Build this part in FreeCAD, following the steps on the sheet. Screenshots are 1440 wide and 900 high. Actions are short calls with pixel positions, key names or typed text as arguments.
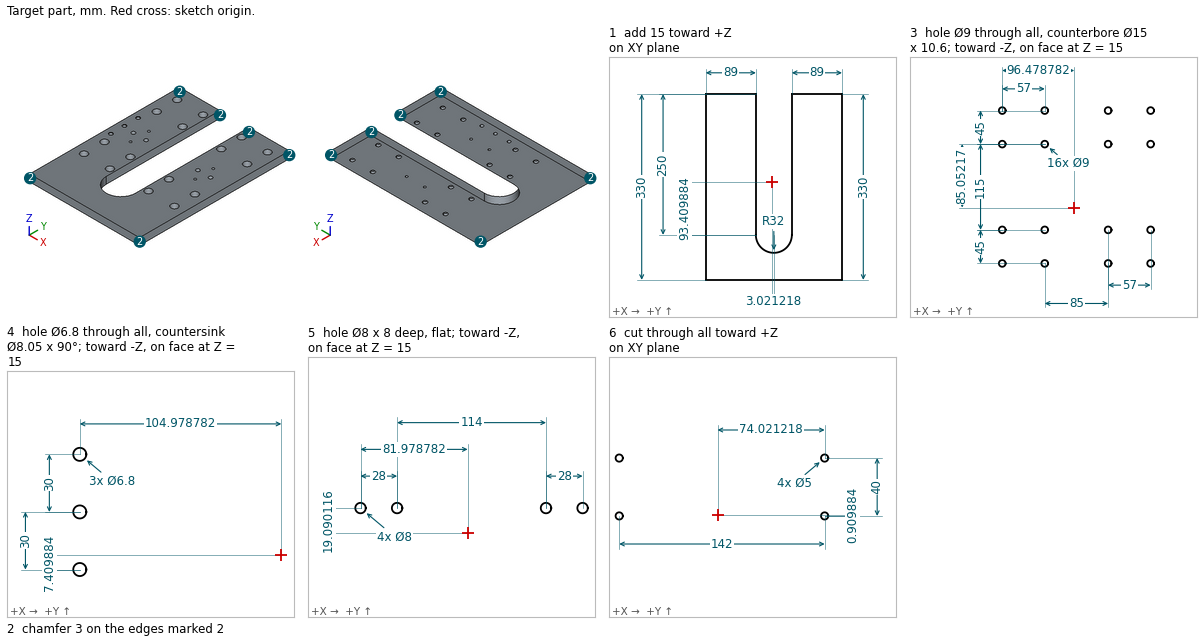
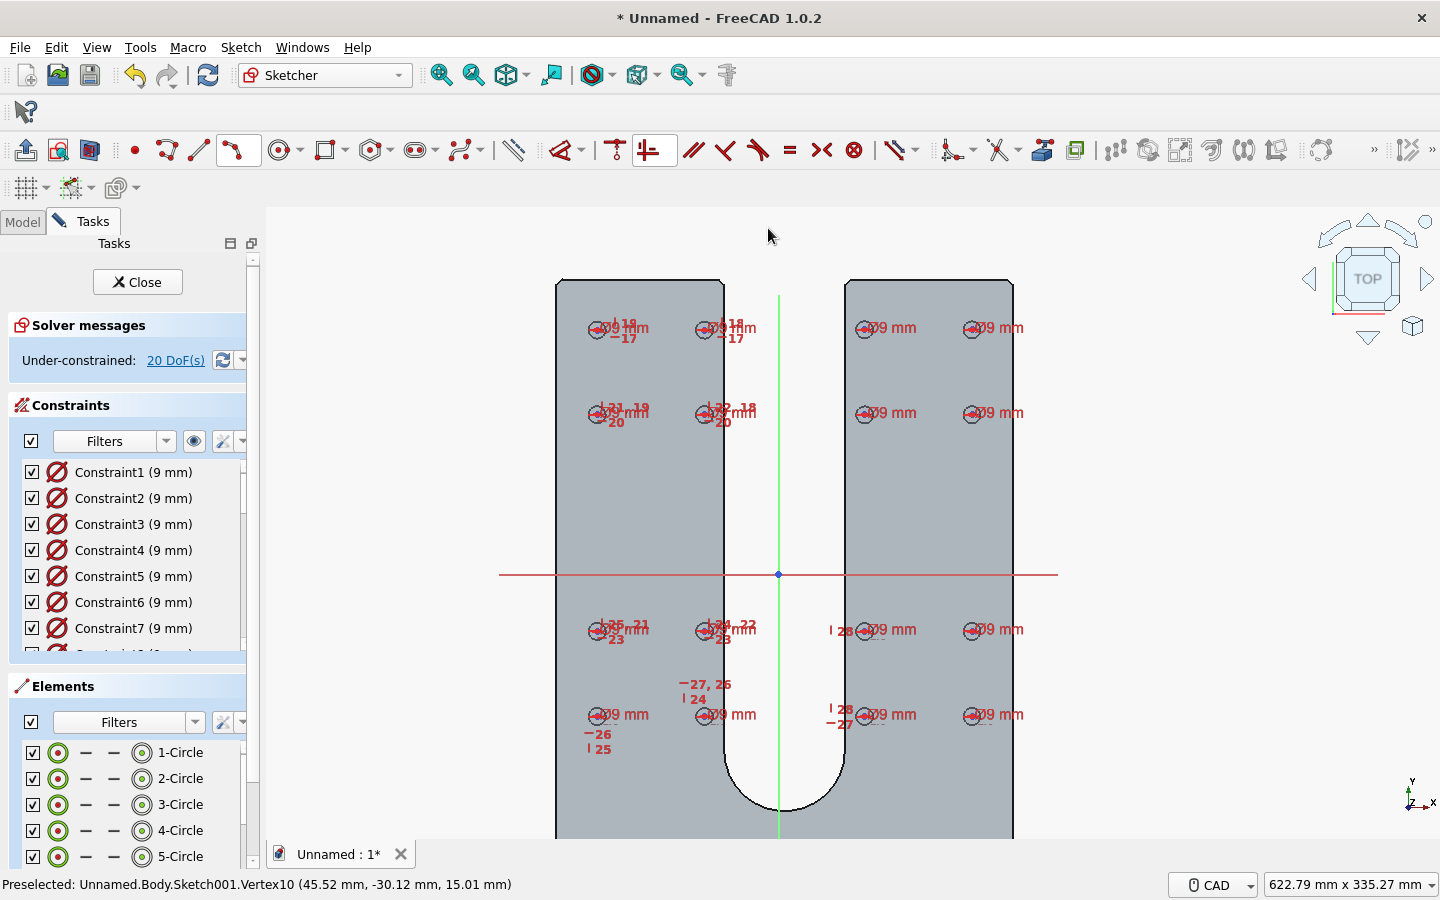
click(705, 631)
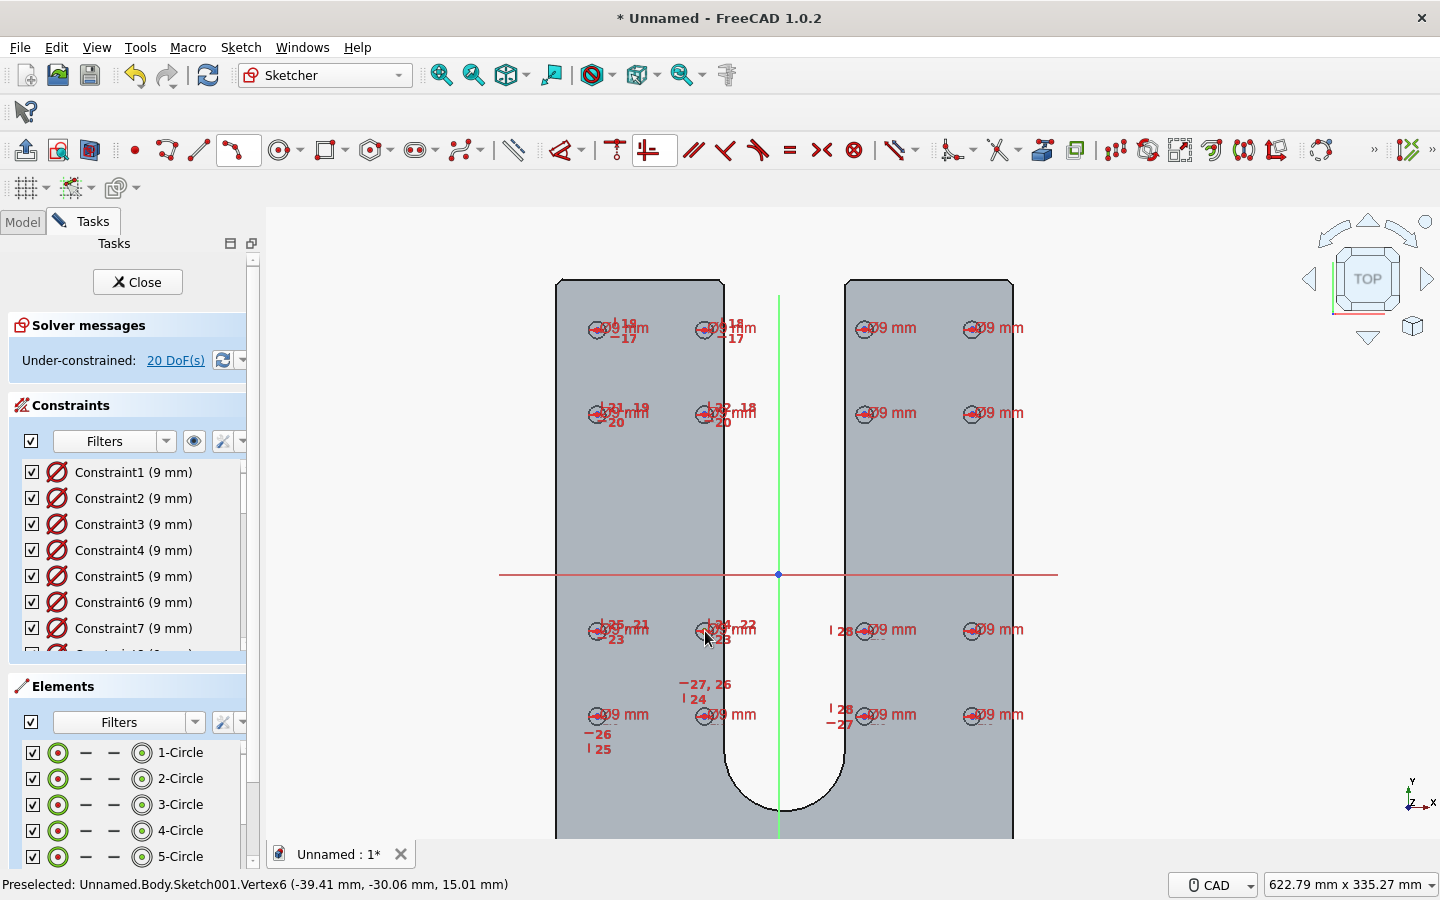
click(865, 632)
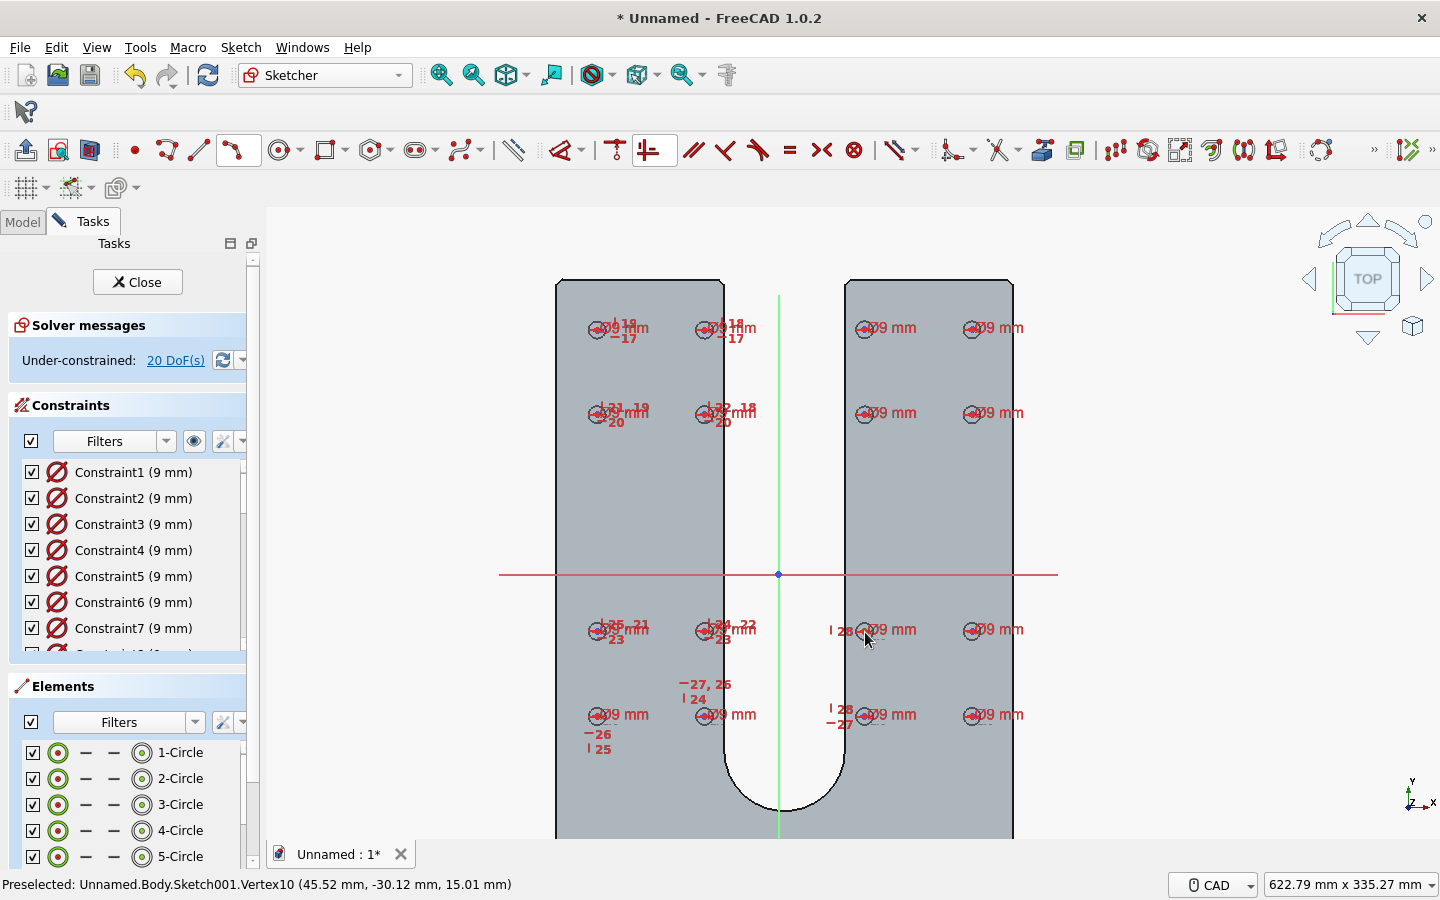
key(h)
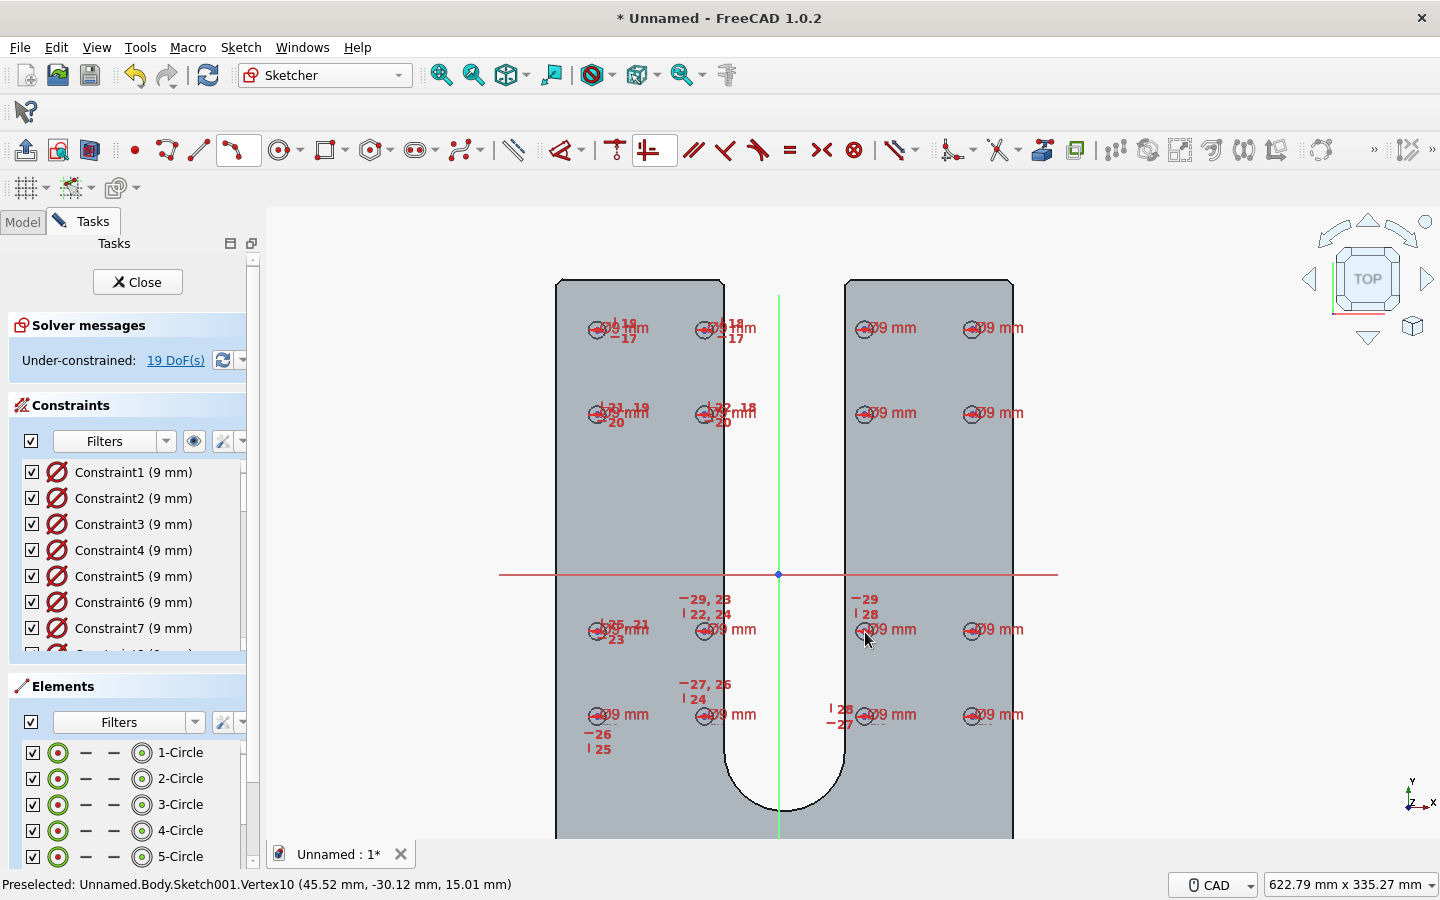
click(865, 631)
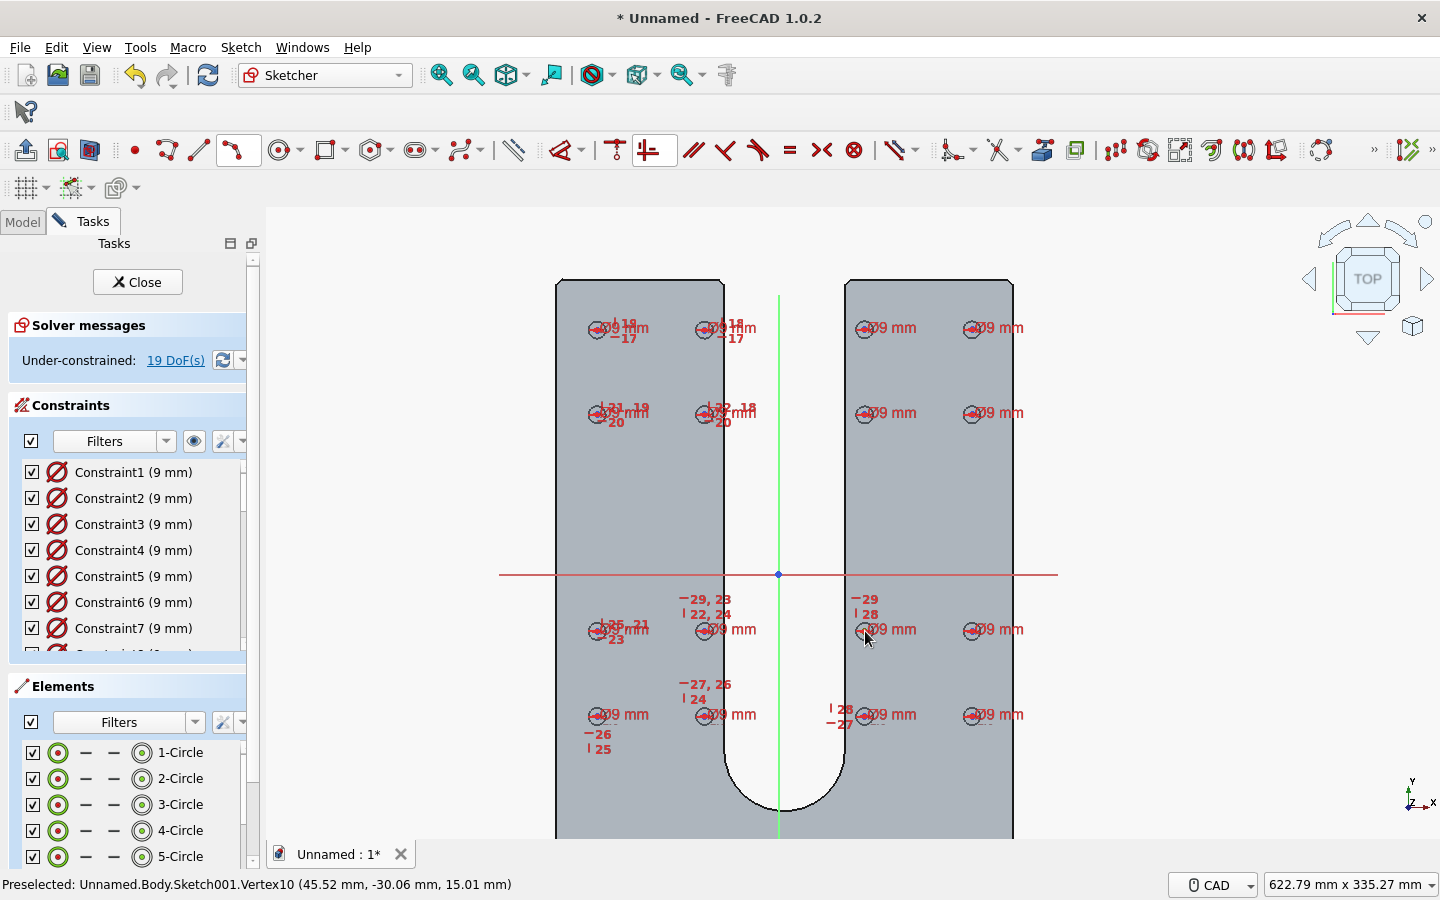
click(972, 631)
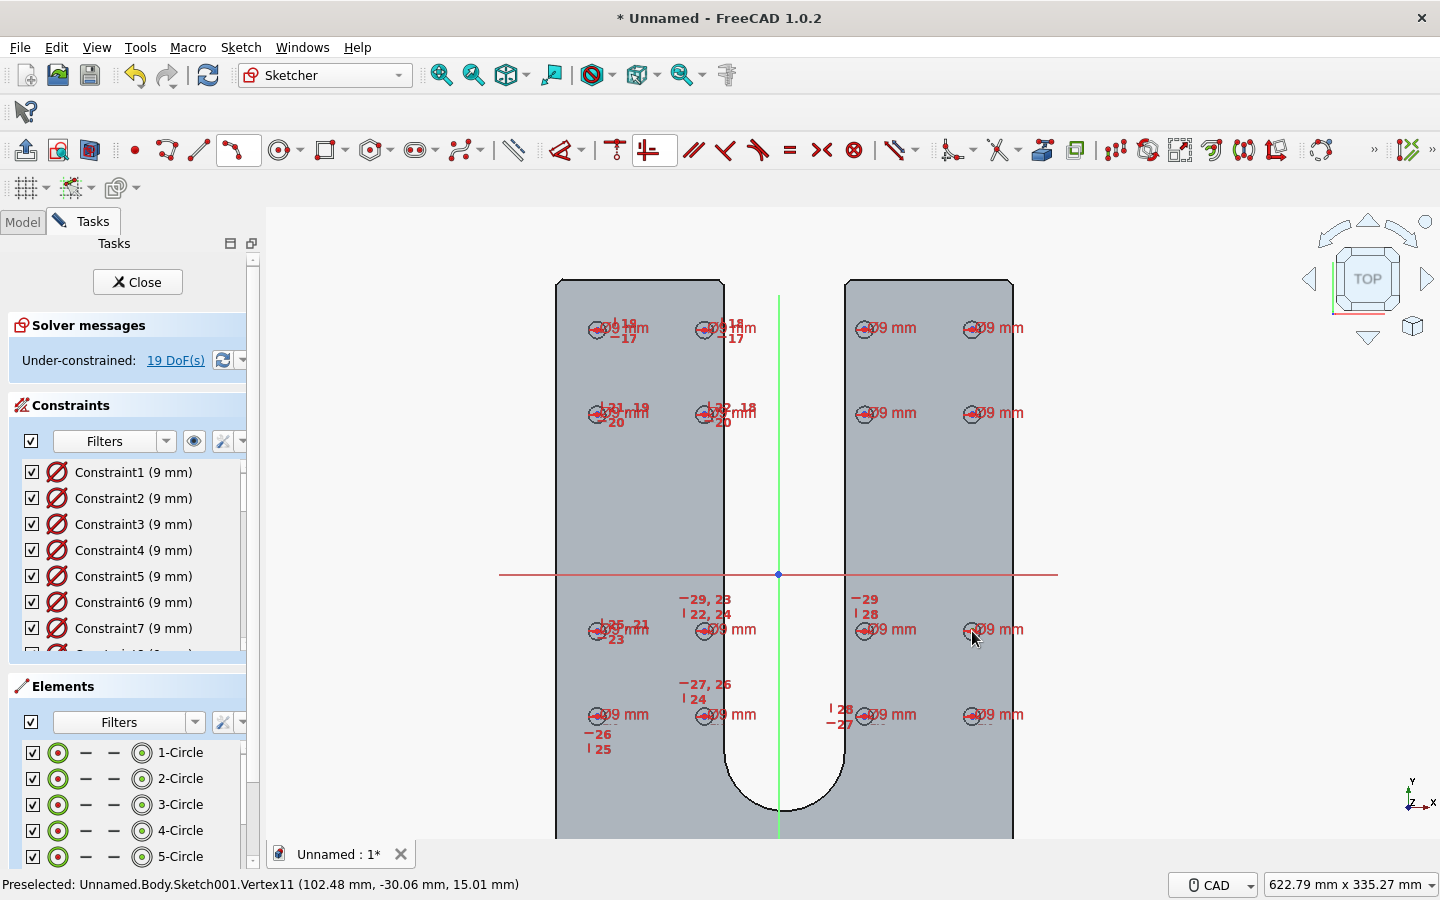
click(672, 150)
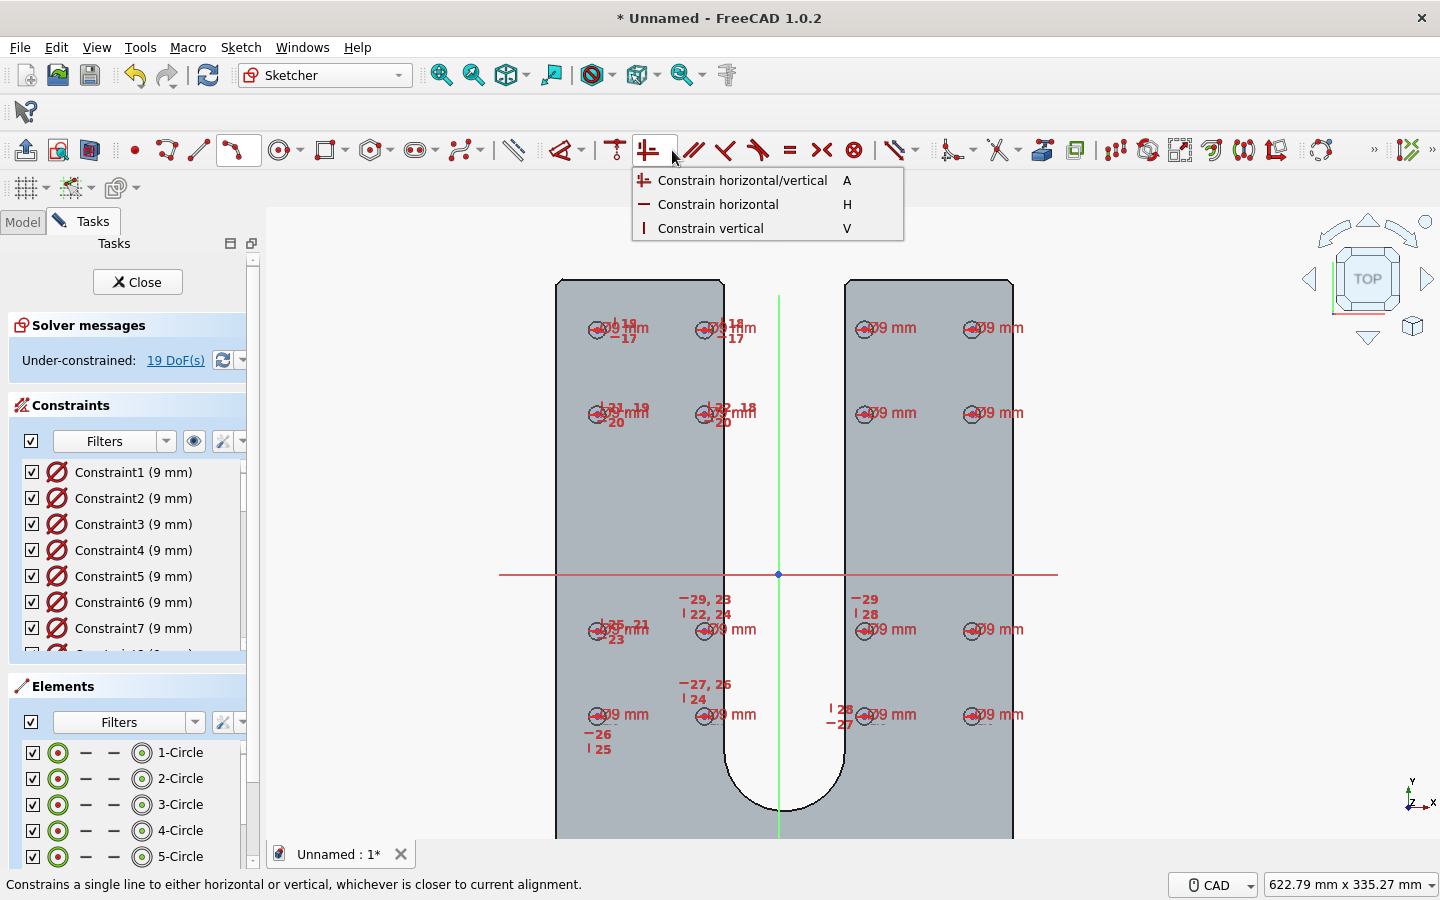
click(768, 204)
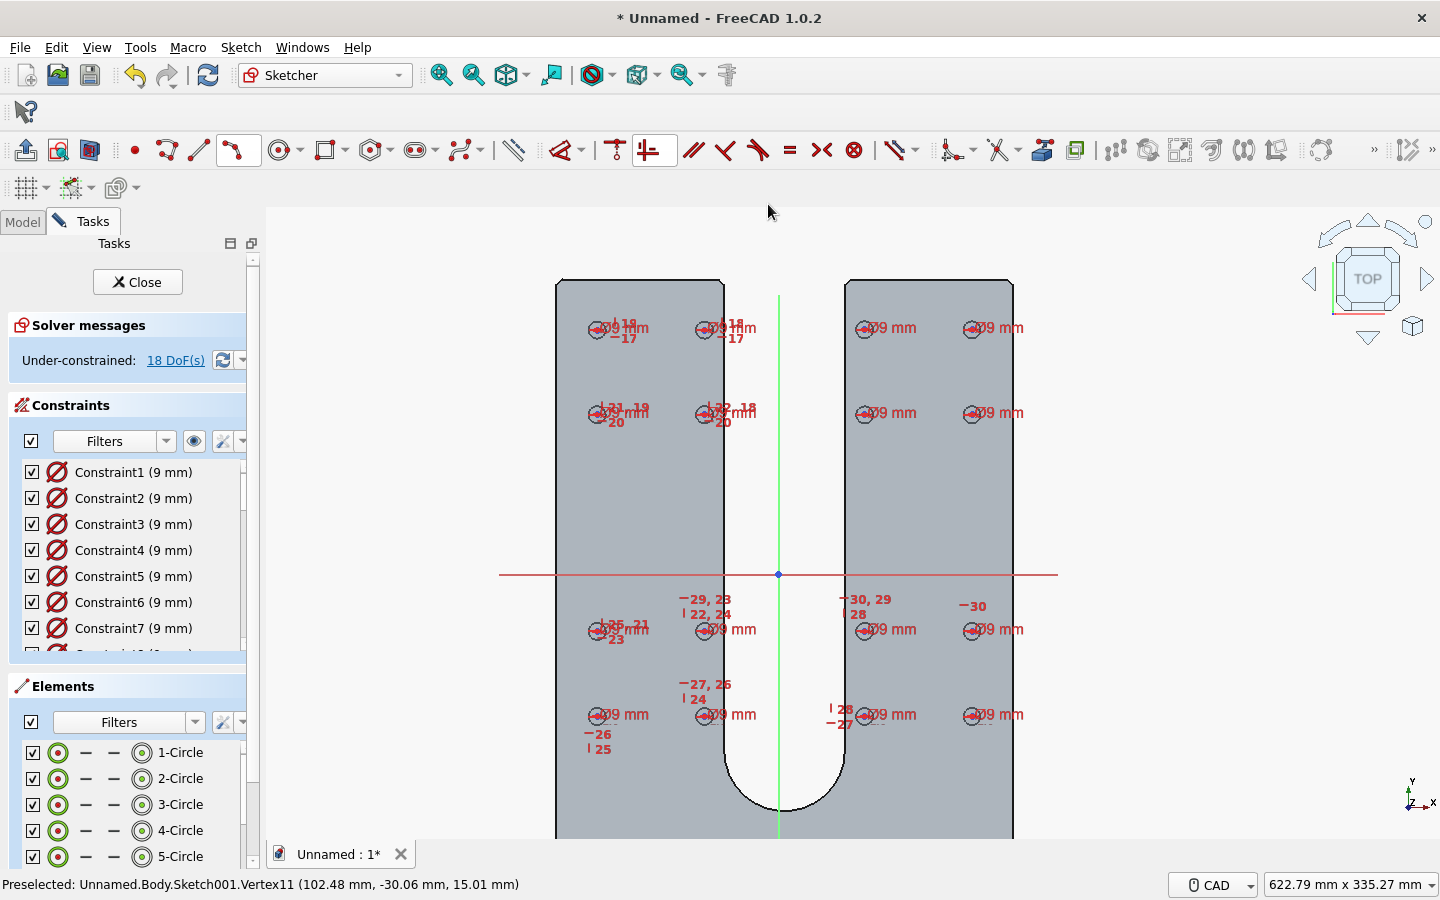
click(972, 631)